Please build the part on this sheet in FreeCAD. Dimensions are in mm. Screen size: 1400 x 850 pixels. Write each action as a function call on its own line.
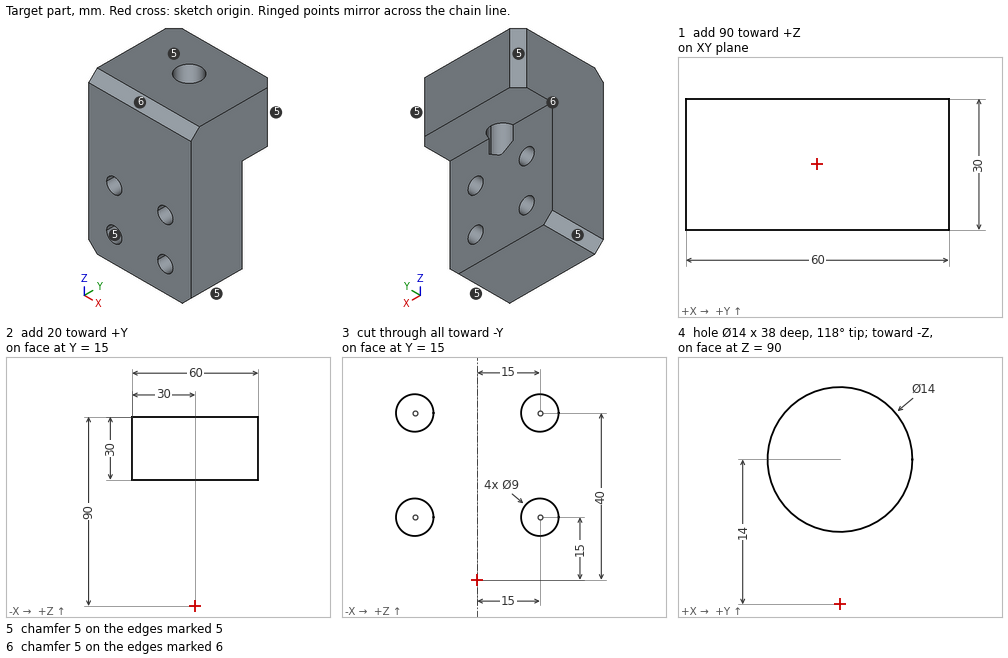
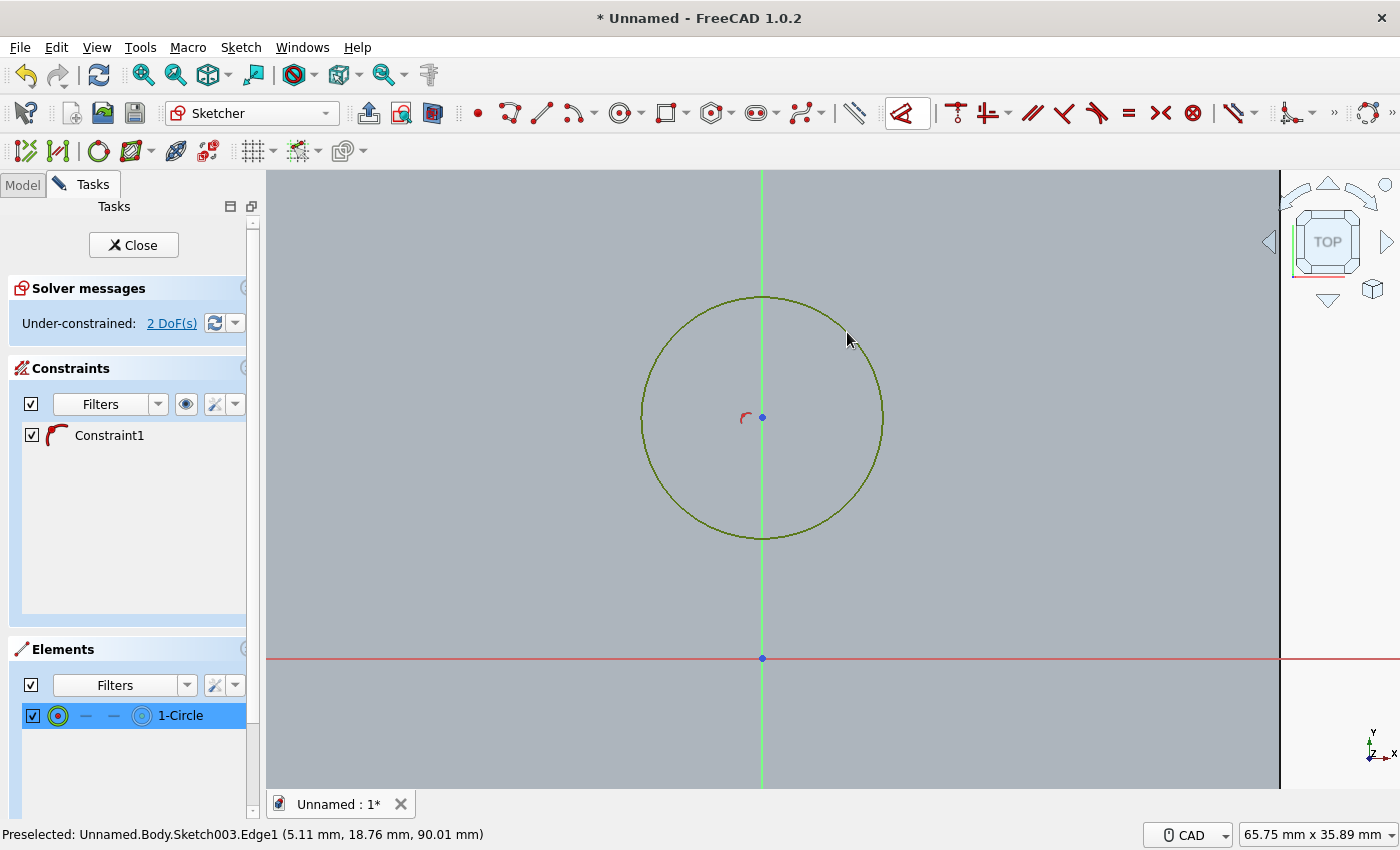
click(924, 114)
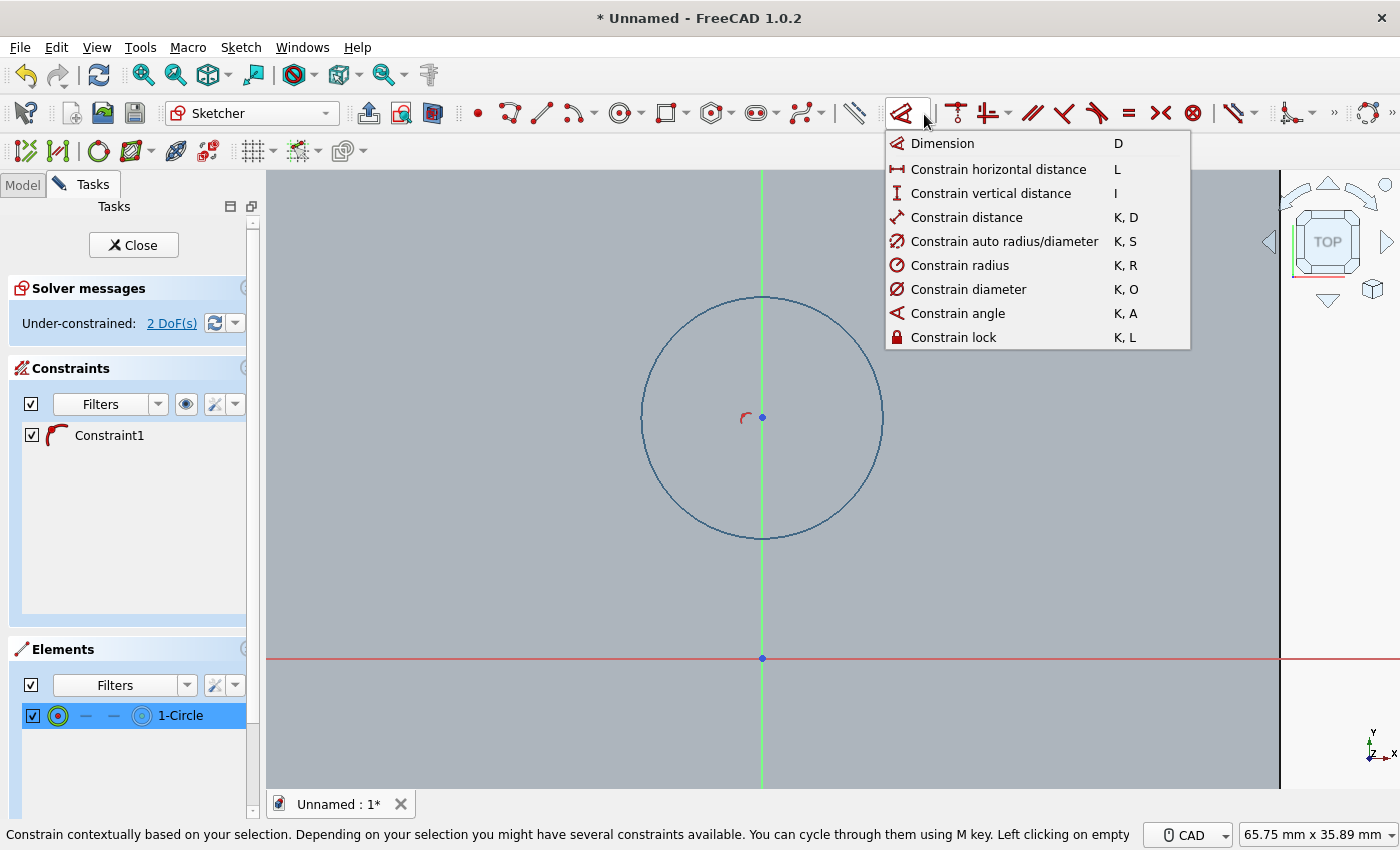
click(1038, 289)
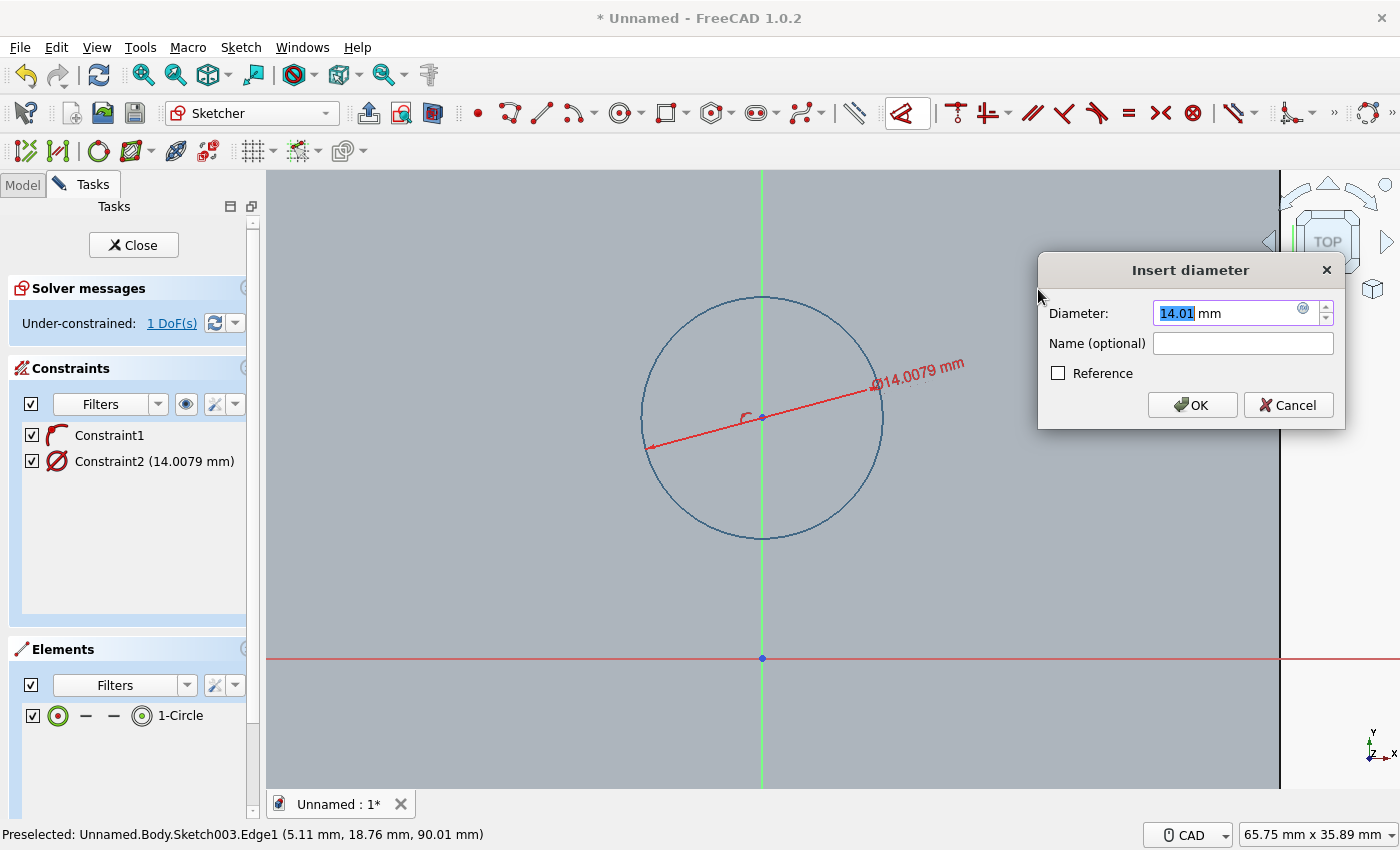
text(14)
key(Return)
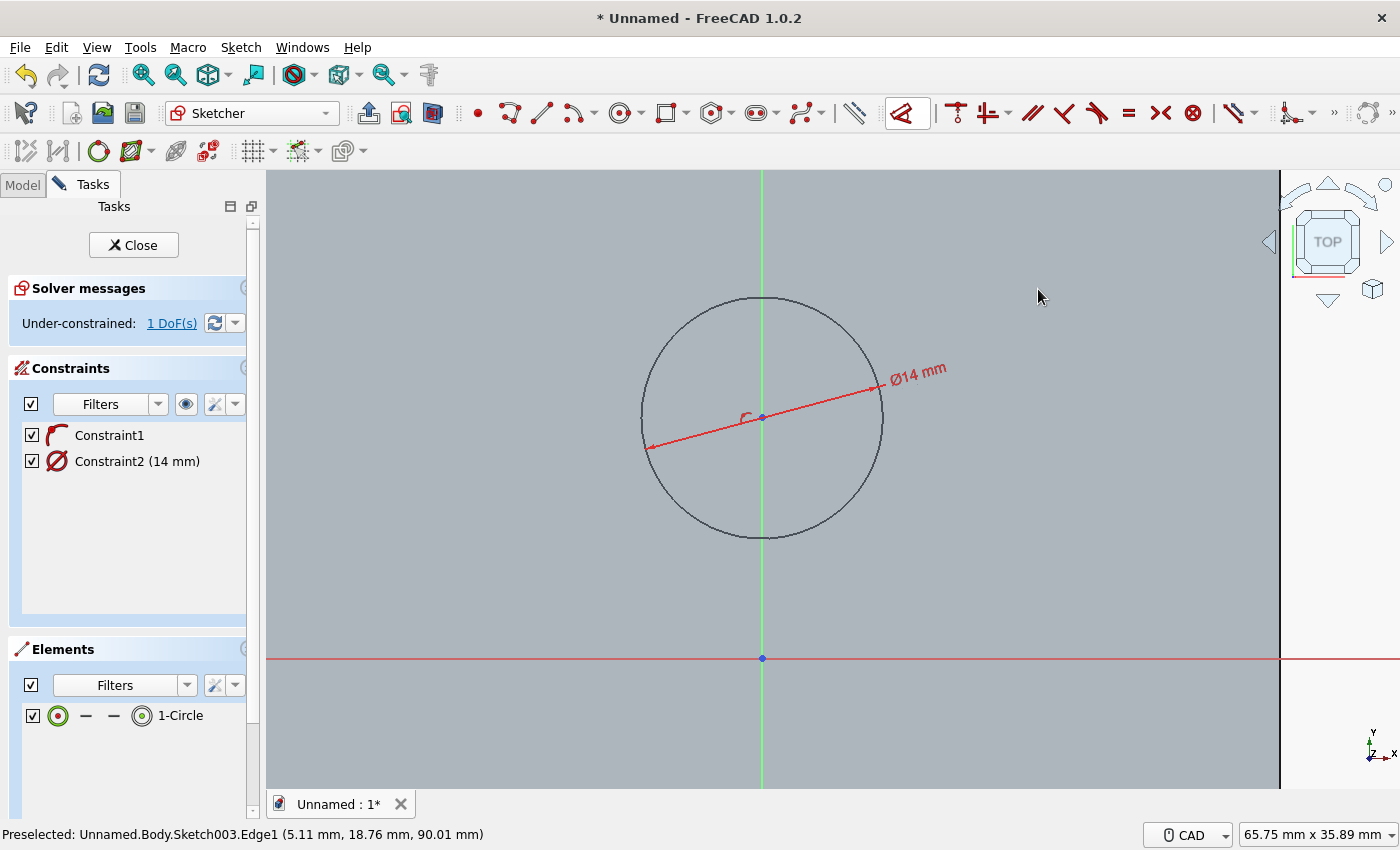
click(762, 418)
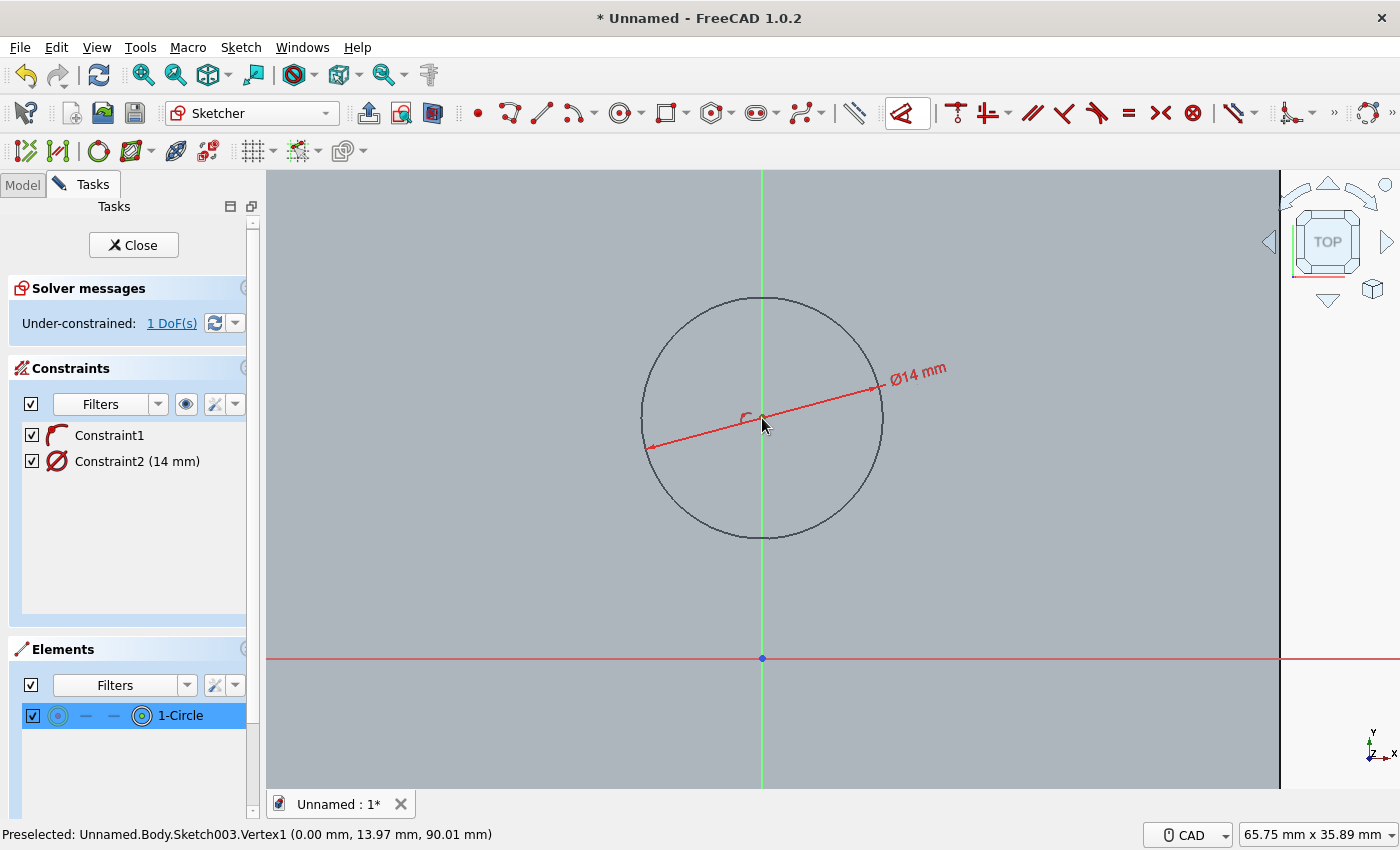
key(i)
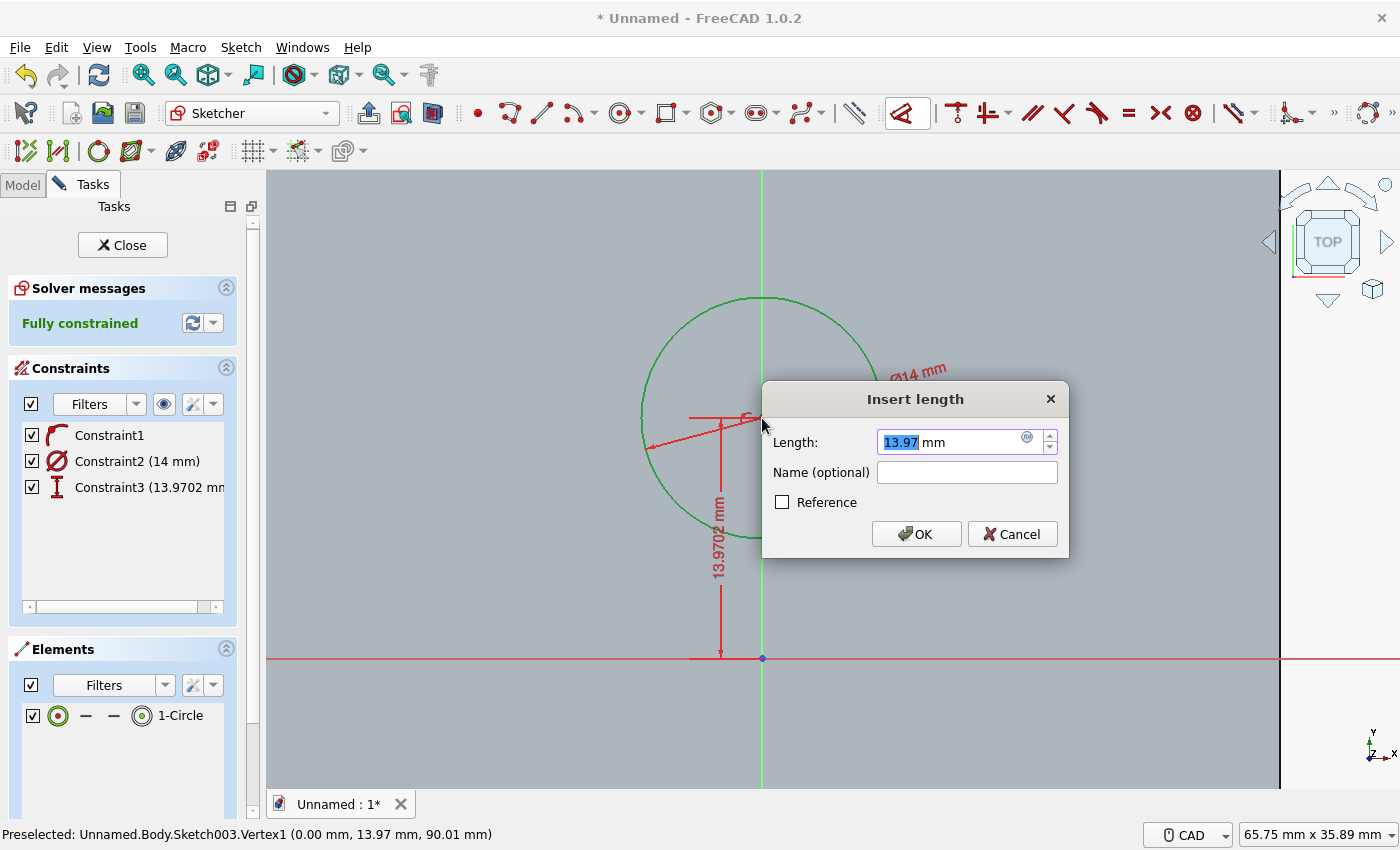
text(14)
key(Return)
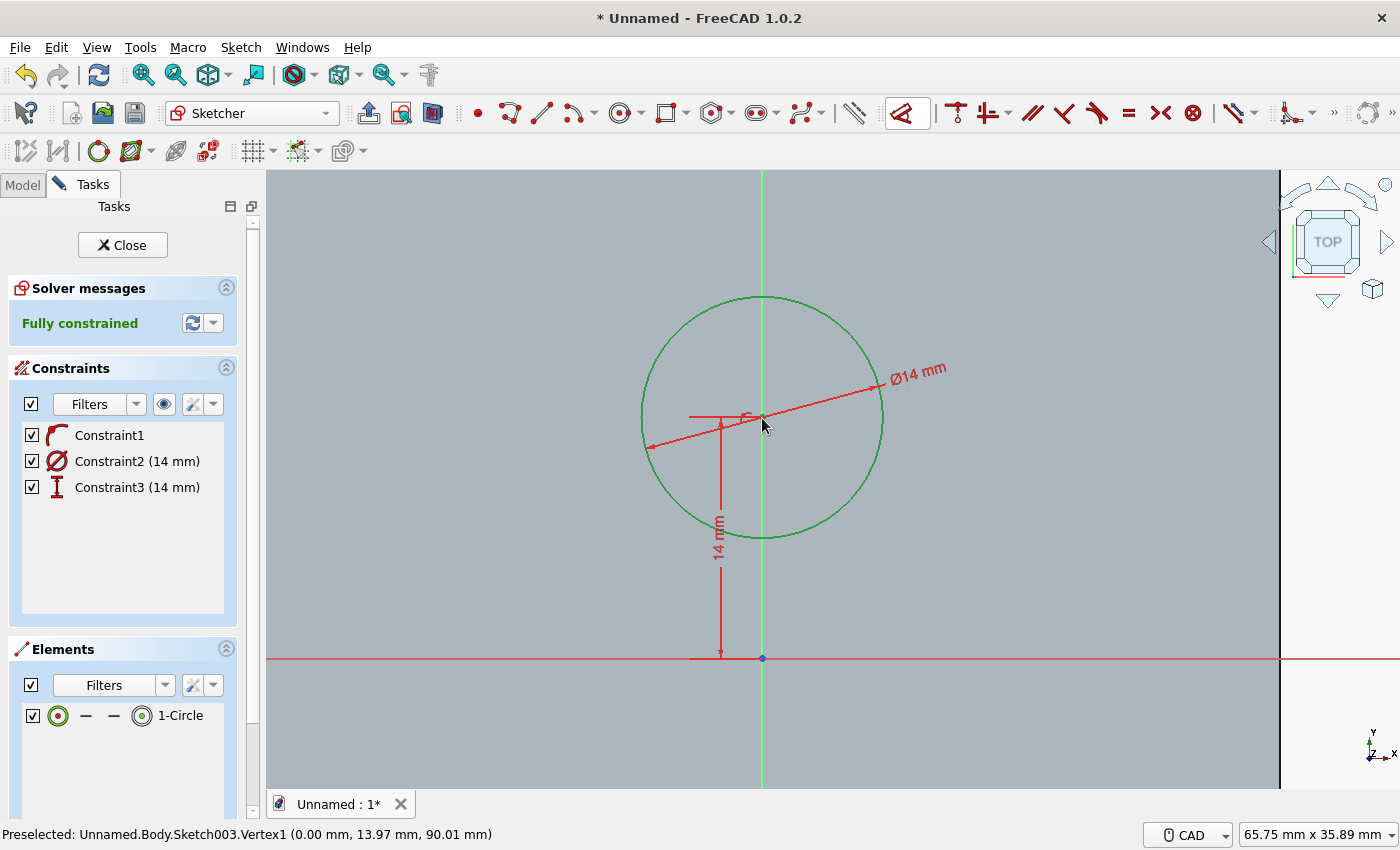
click(123, 245)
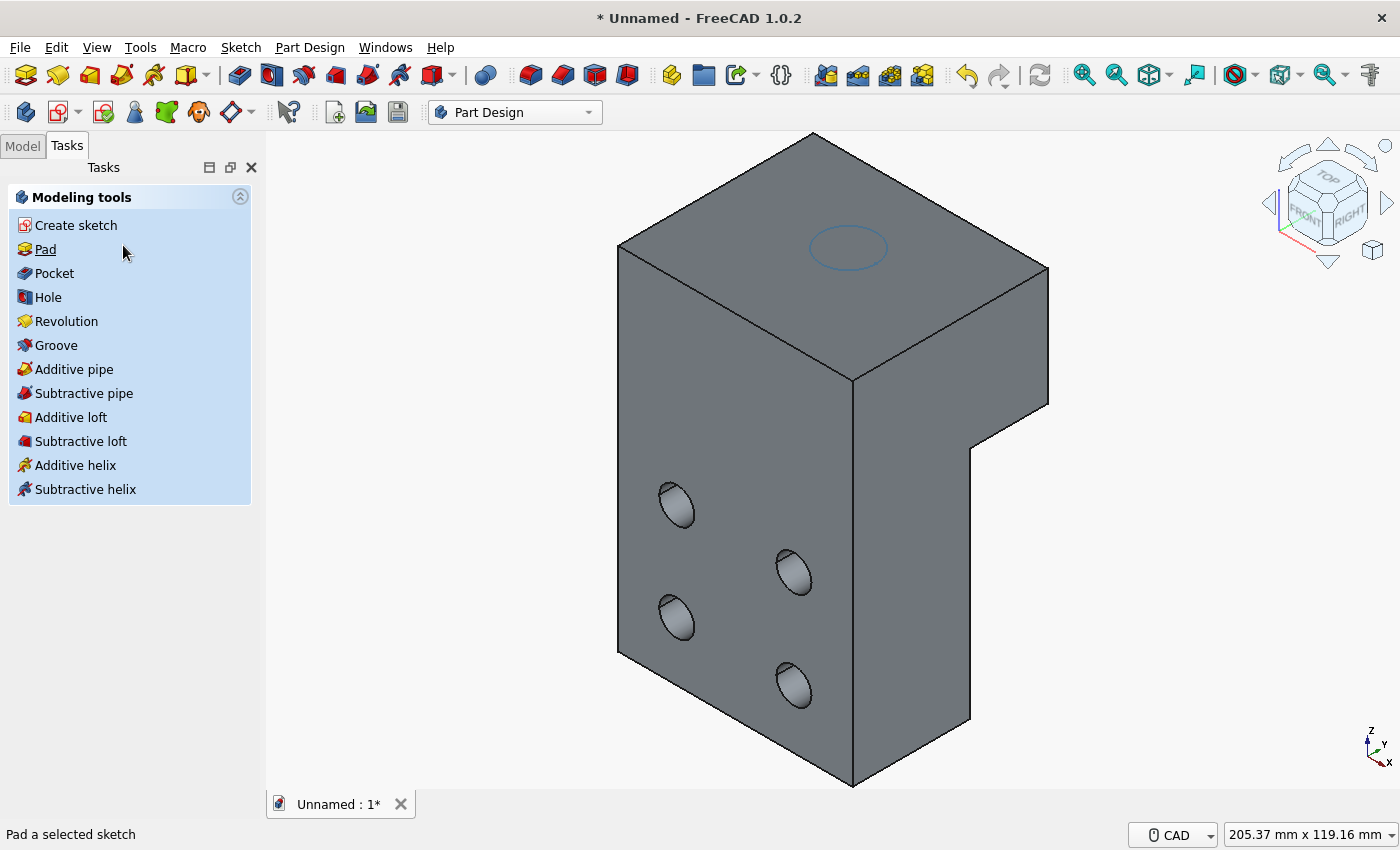
click(272, 76)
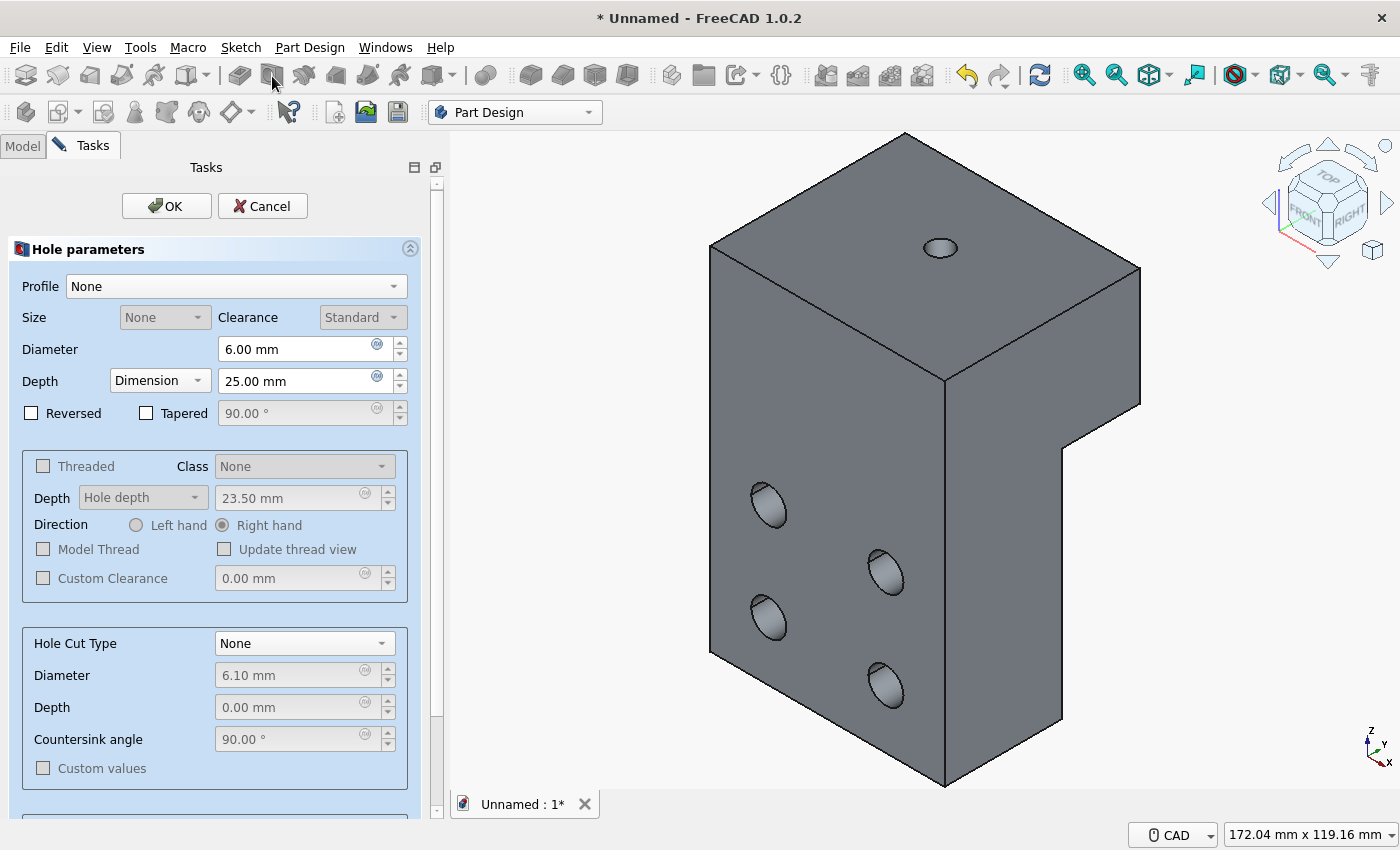
triple_click(305, 349)